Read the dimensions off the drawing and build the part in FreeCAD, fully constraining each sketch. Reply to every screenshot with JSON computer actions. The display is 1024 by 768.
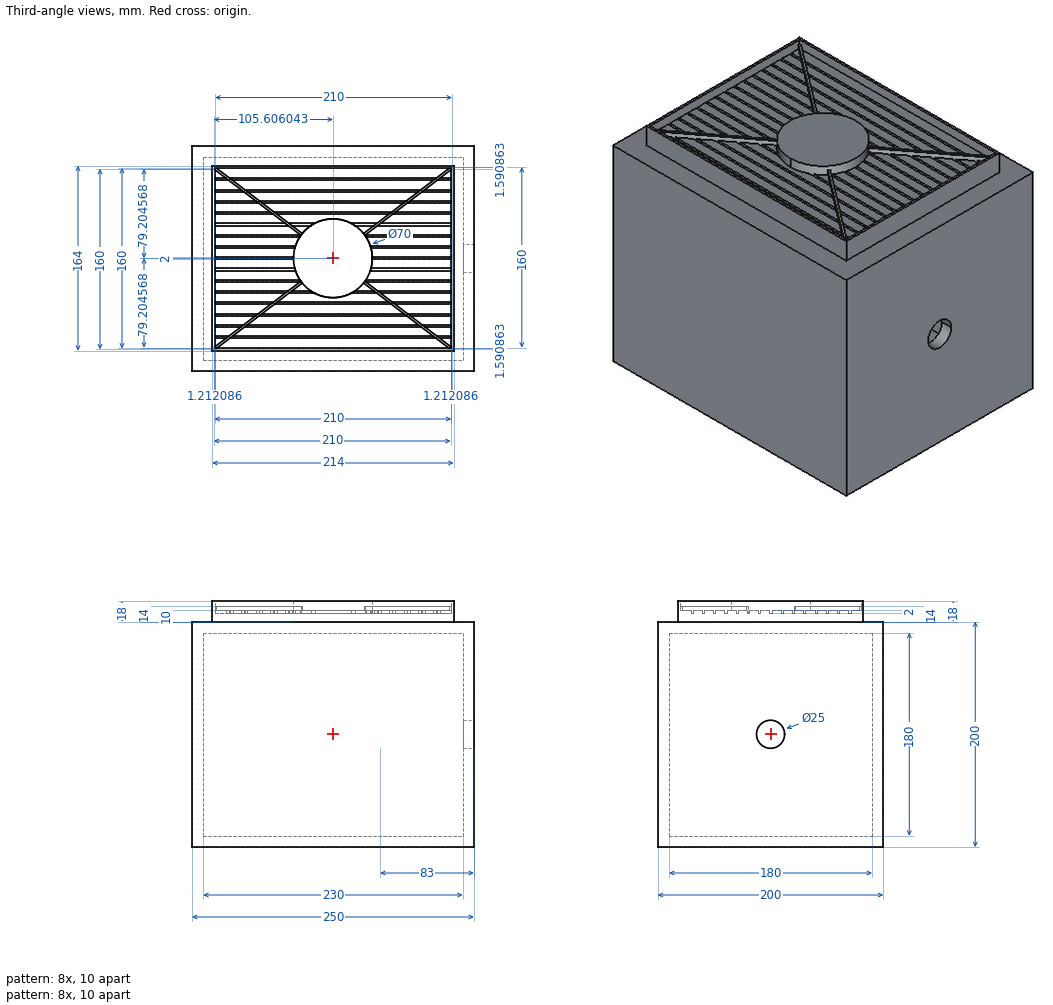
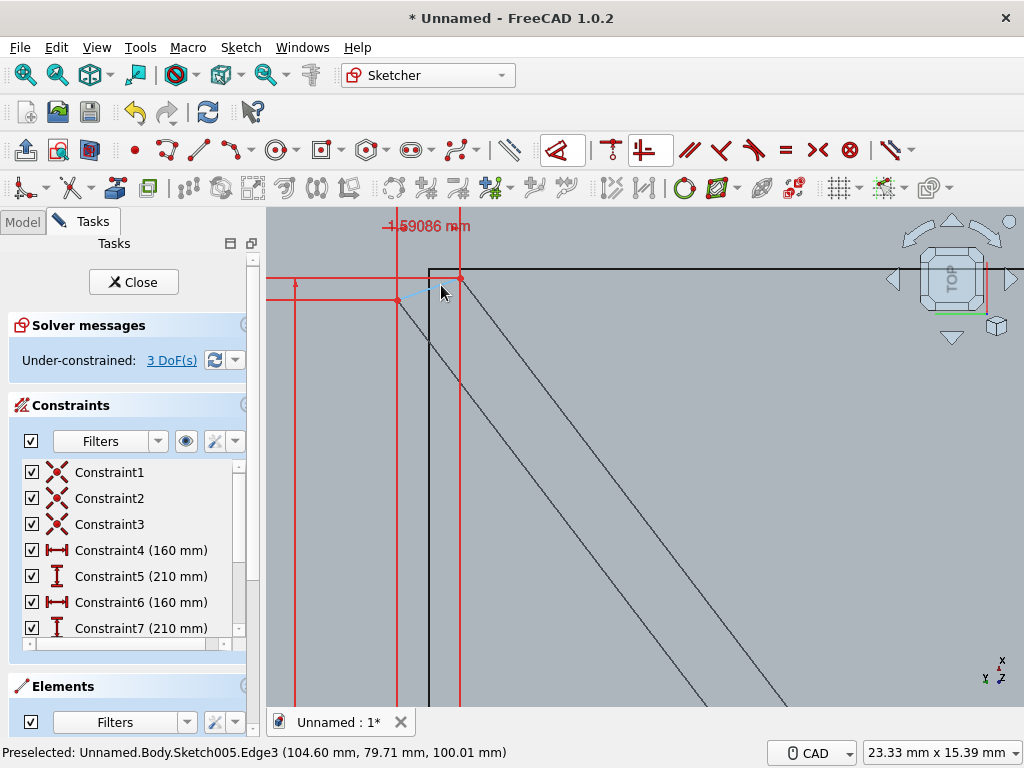
{"action": "left_click", "coordinate": [442, 285]}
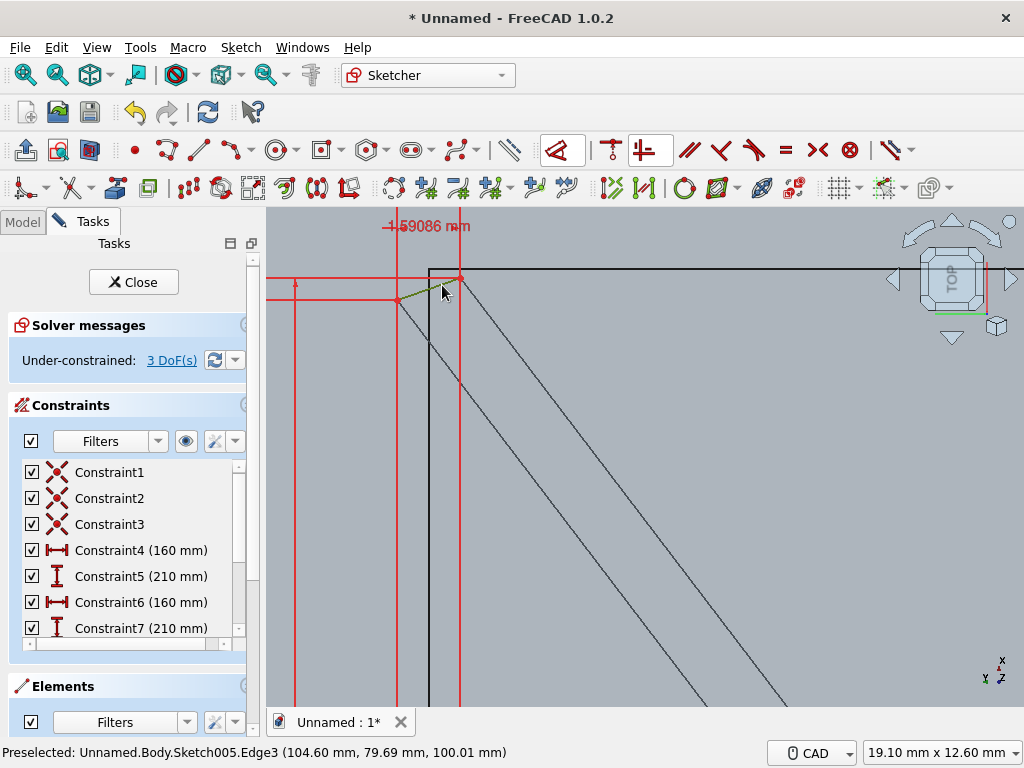
{"action": "key", "text": "i"}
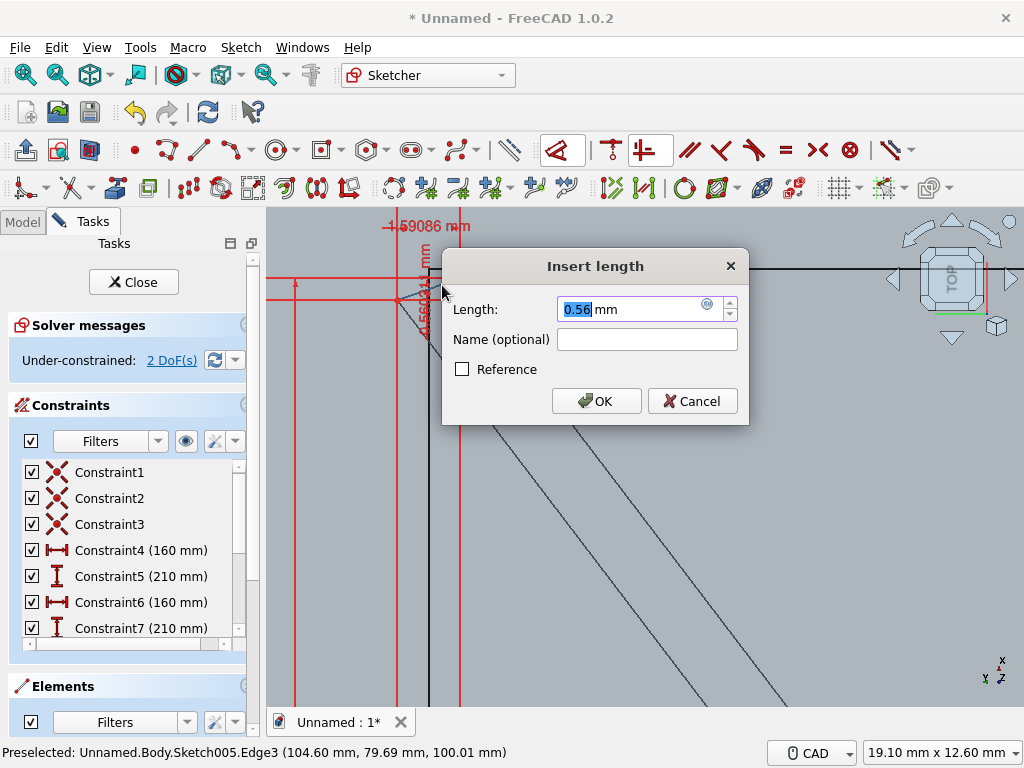
{"action": "type", "text": "1.212086"}
{"action": "key", "text": "Return"}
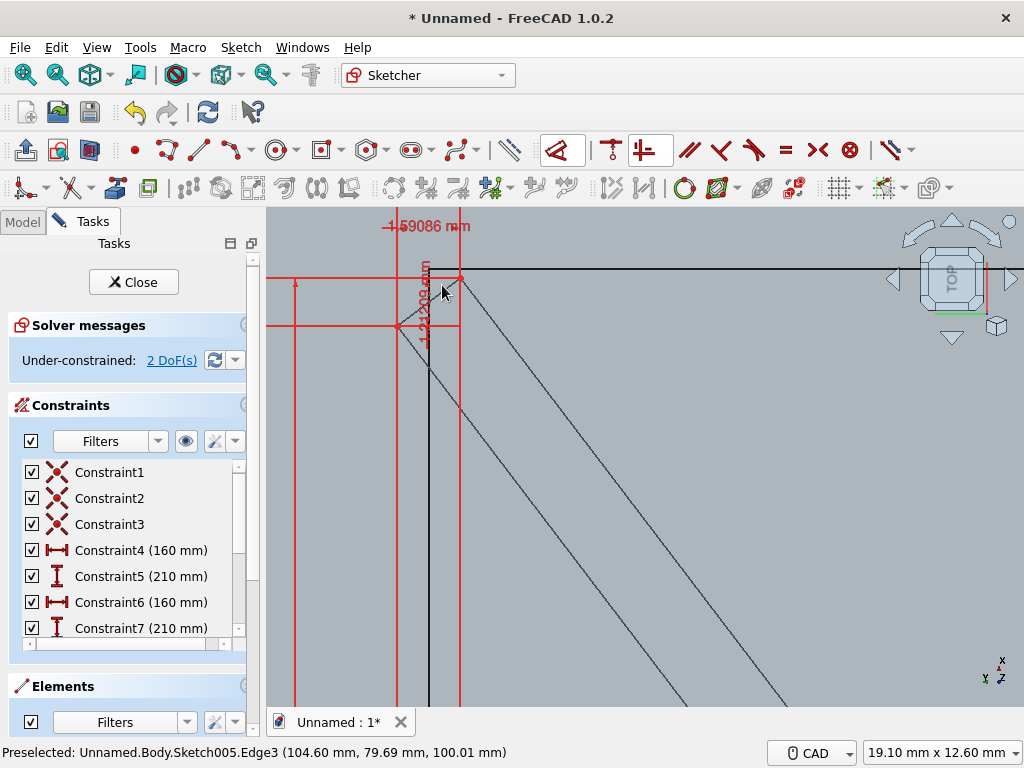
{"action": "scroll", "coordinate": [448, 288], "scroll_direction": "down", "scroll_amount": 16}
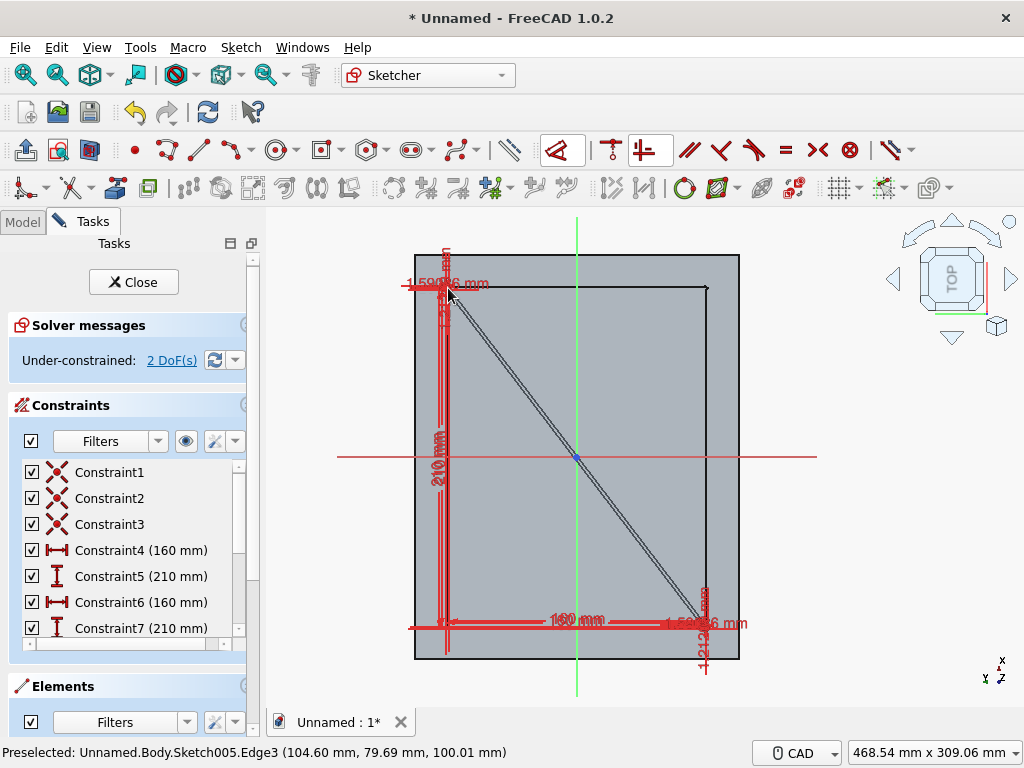
{"action": "scroll", "coordinate": [705, 629], "scroll_direction": "up", "scroll_amount": 7}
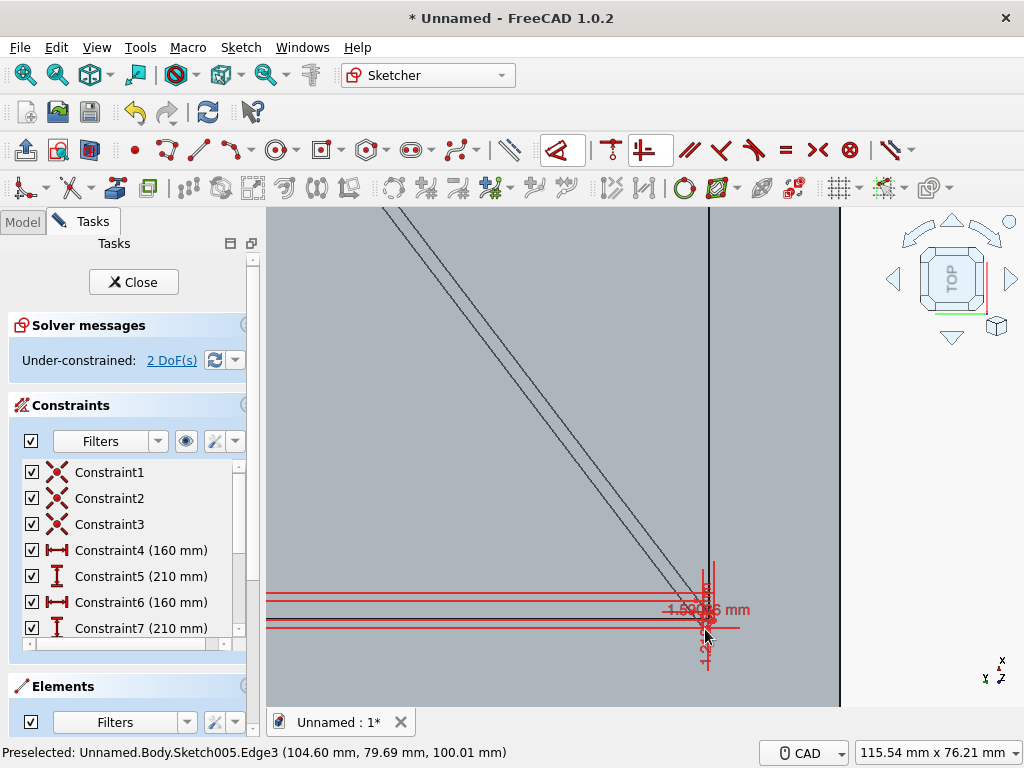
{"action": "left_click", "coordinate": [703, 628]}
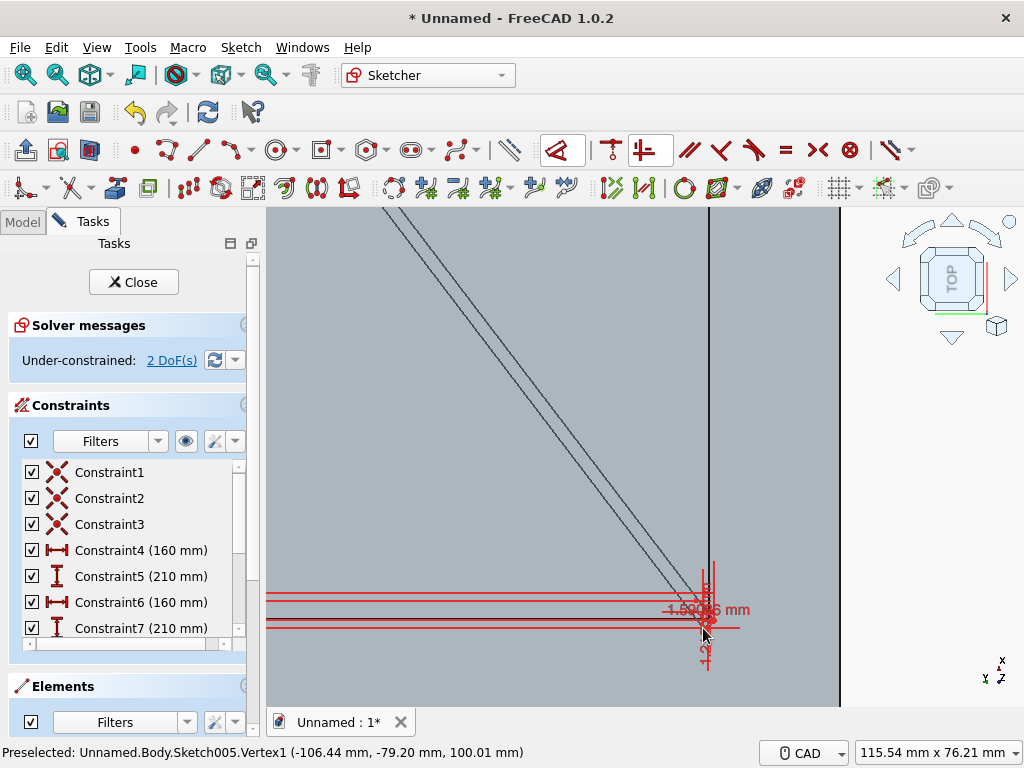
{"action": "left_click", "coordinate": [580, 150]}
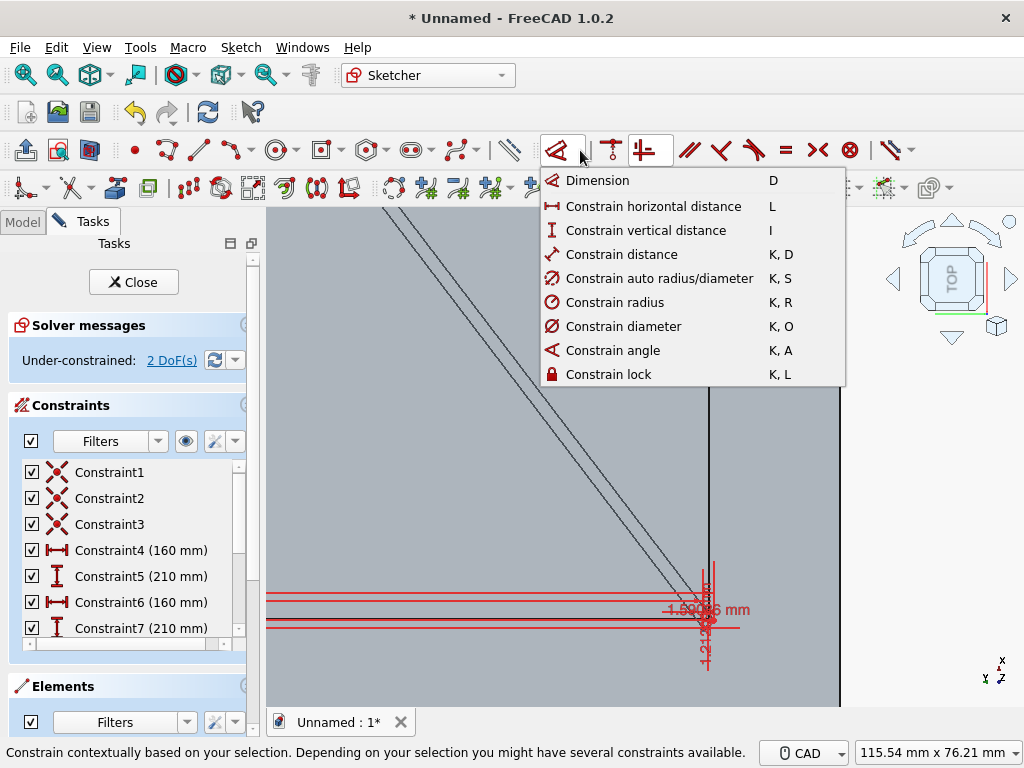
{"action": "left_click", "coordinate": [693, 206]}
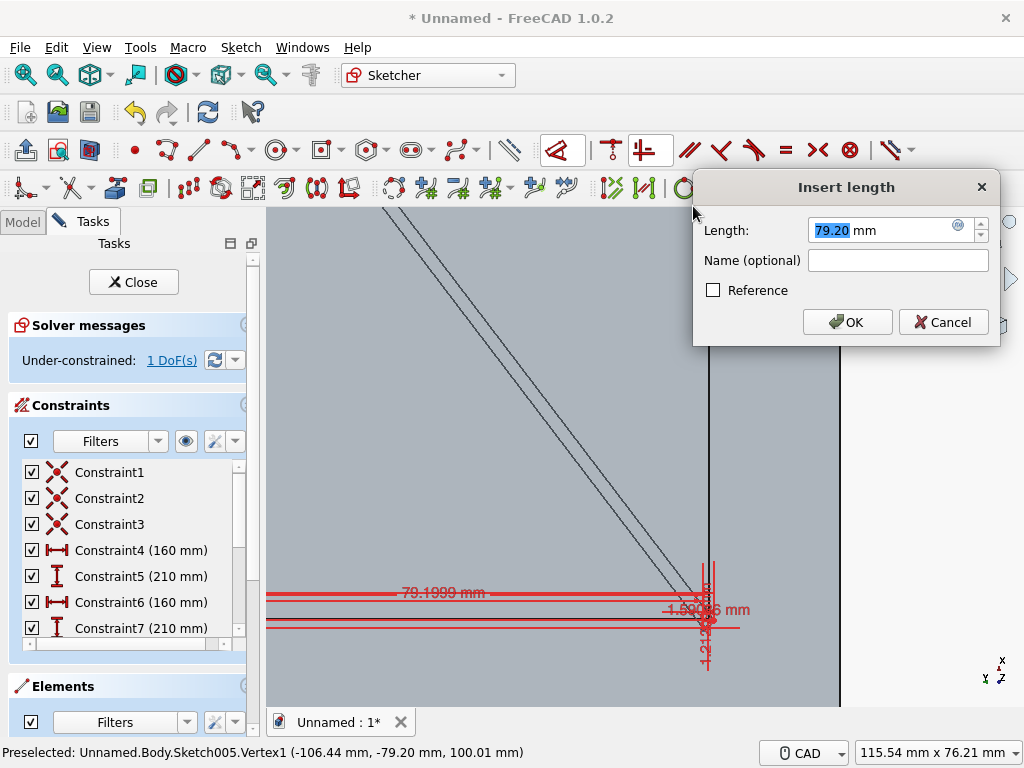
{"action": "type", "text": "79.204568"}
{"action": "key", "text": "Return"}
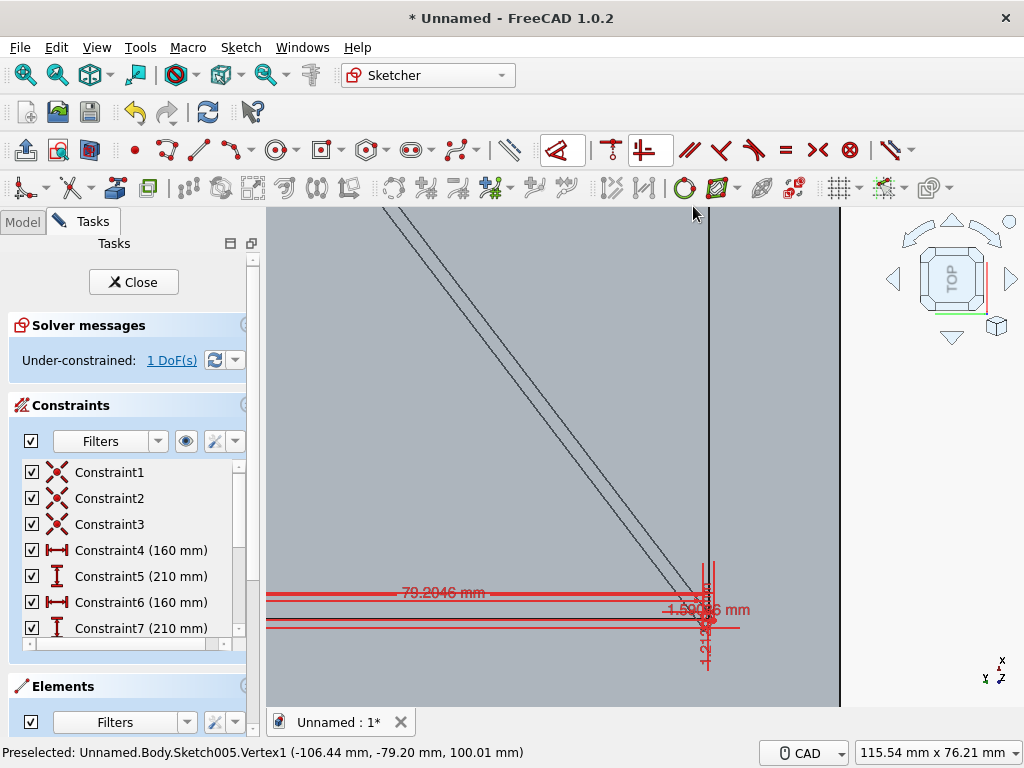
{"action": "left_click", "coordinate": [703, 628]}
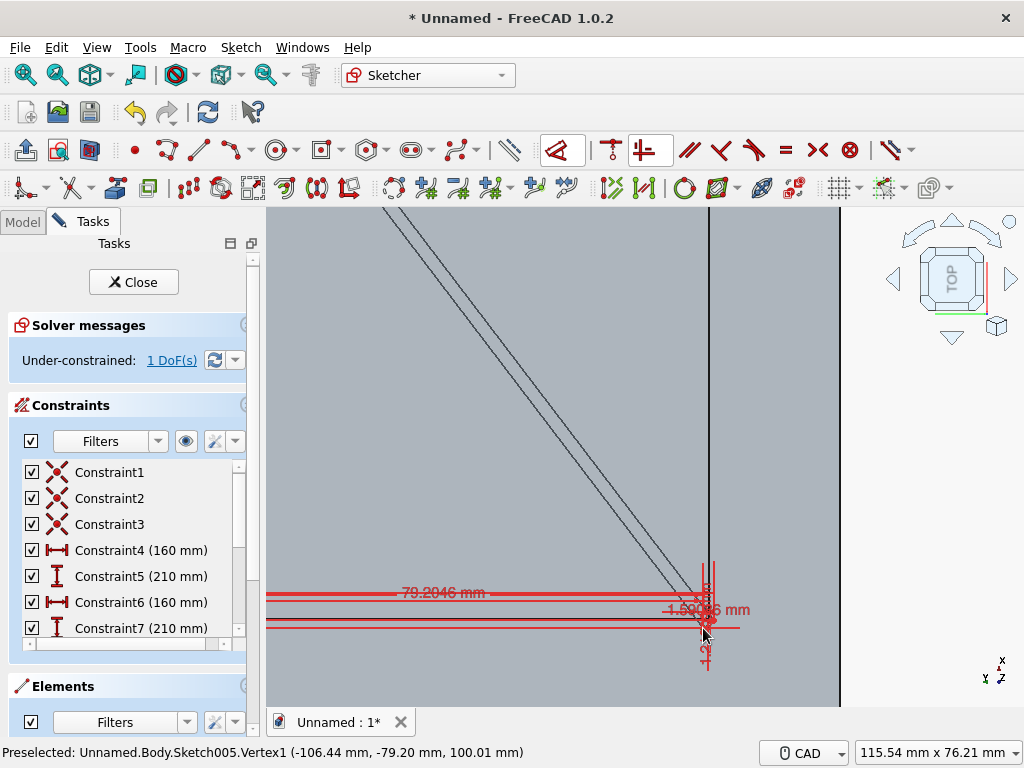
{"action": "key", "text": "i"}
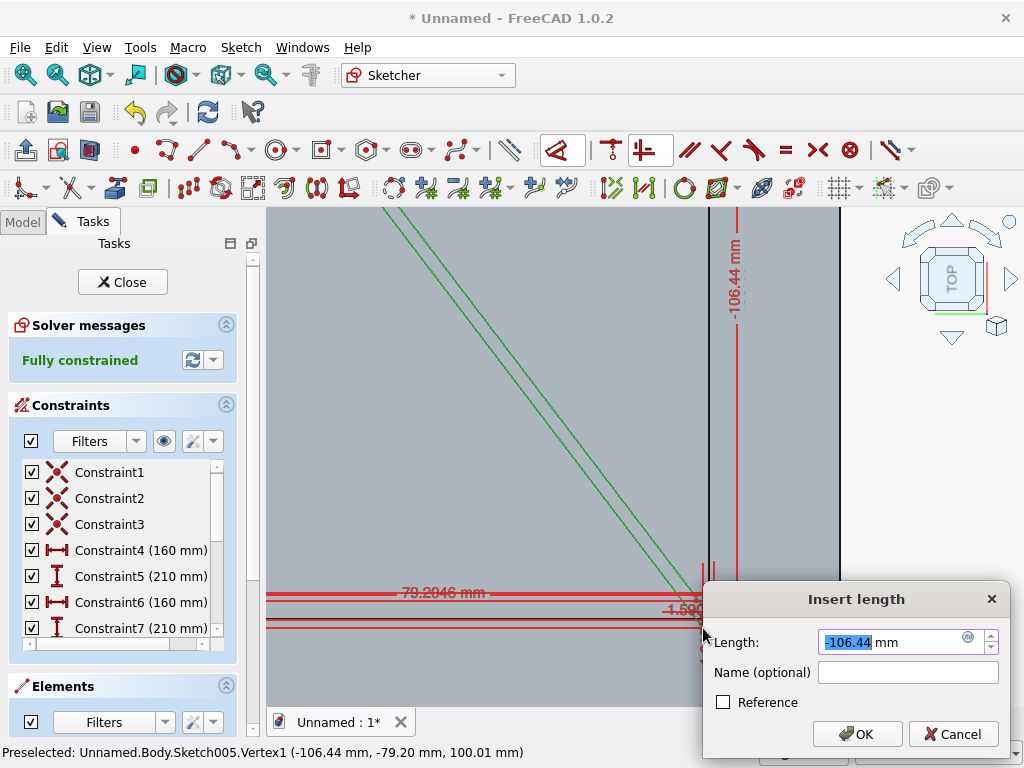
{"action": "type", "text": "-105.606043"}
{"action": "key", "text": "Return"}